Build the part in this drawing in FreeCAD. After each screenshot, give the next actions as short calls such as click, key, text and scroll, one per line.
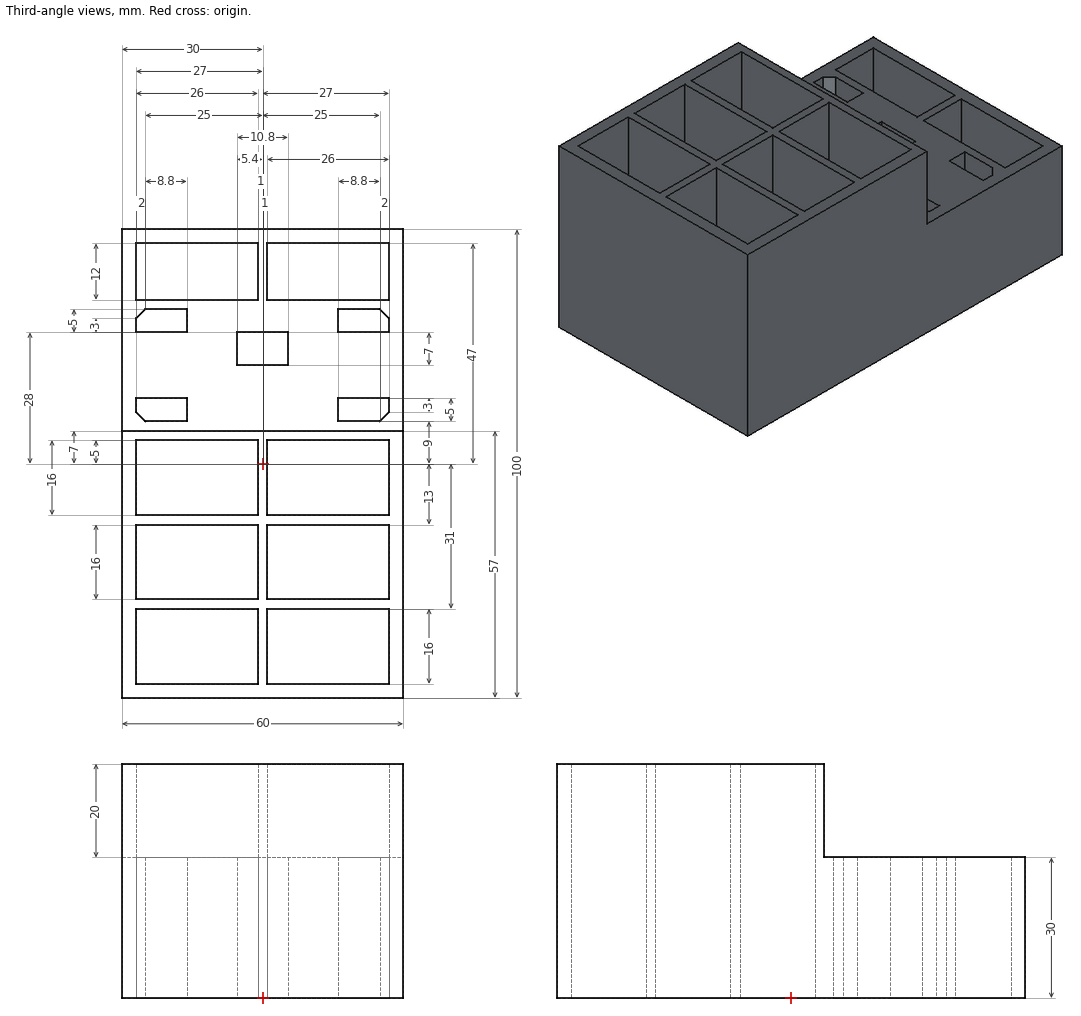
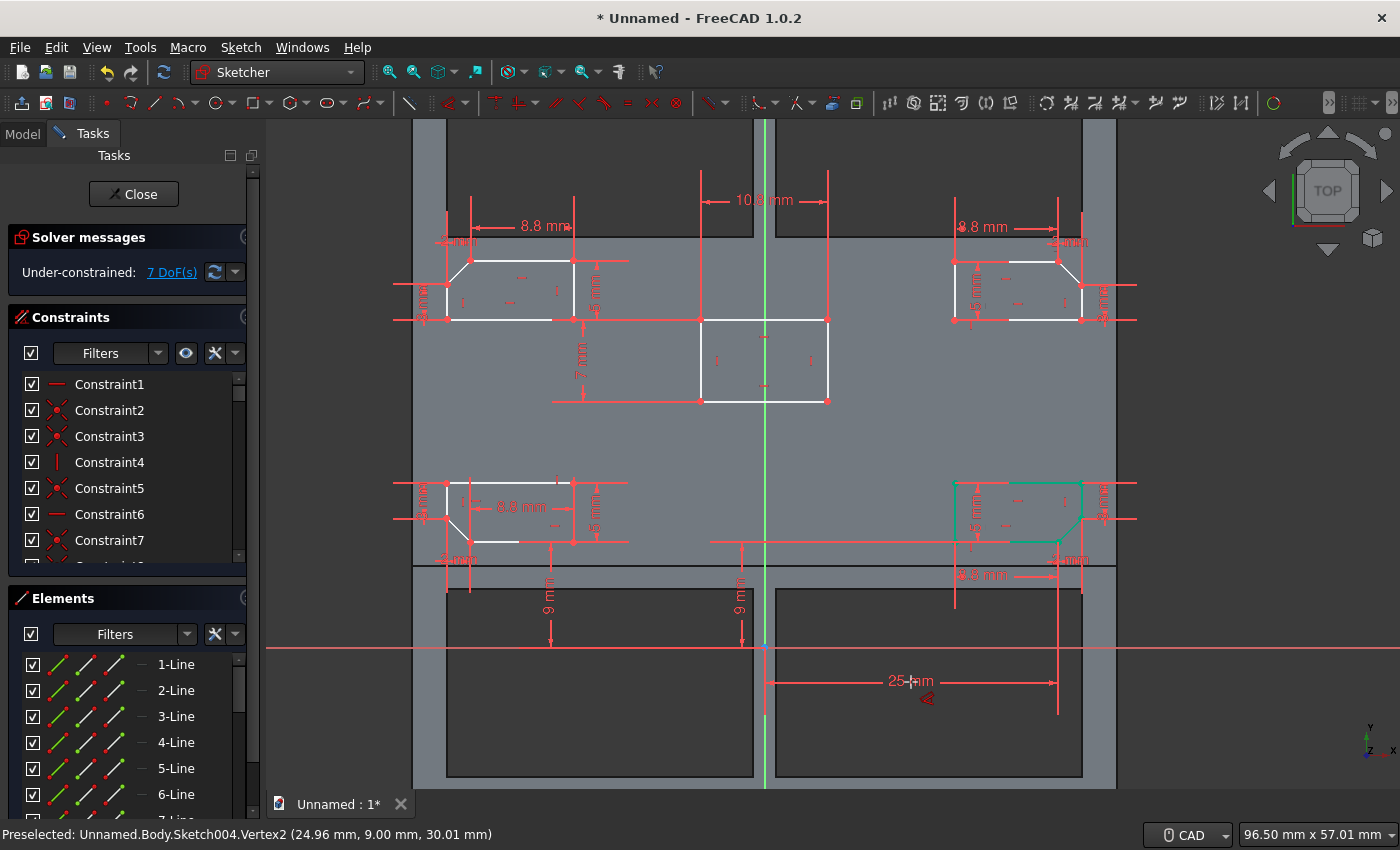
click(701, 320)
click(667, 484)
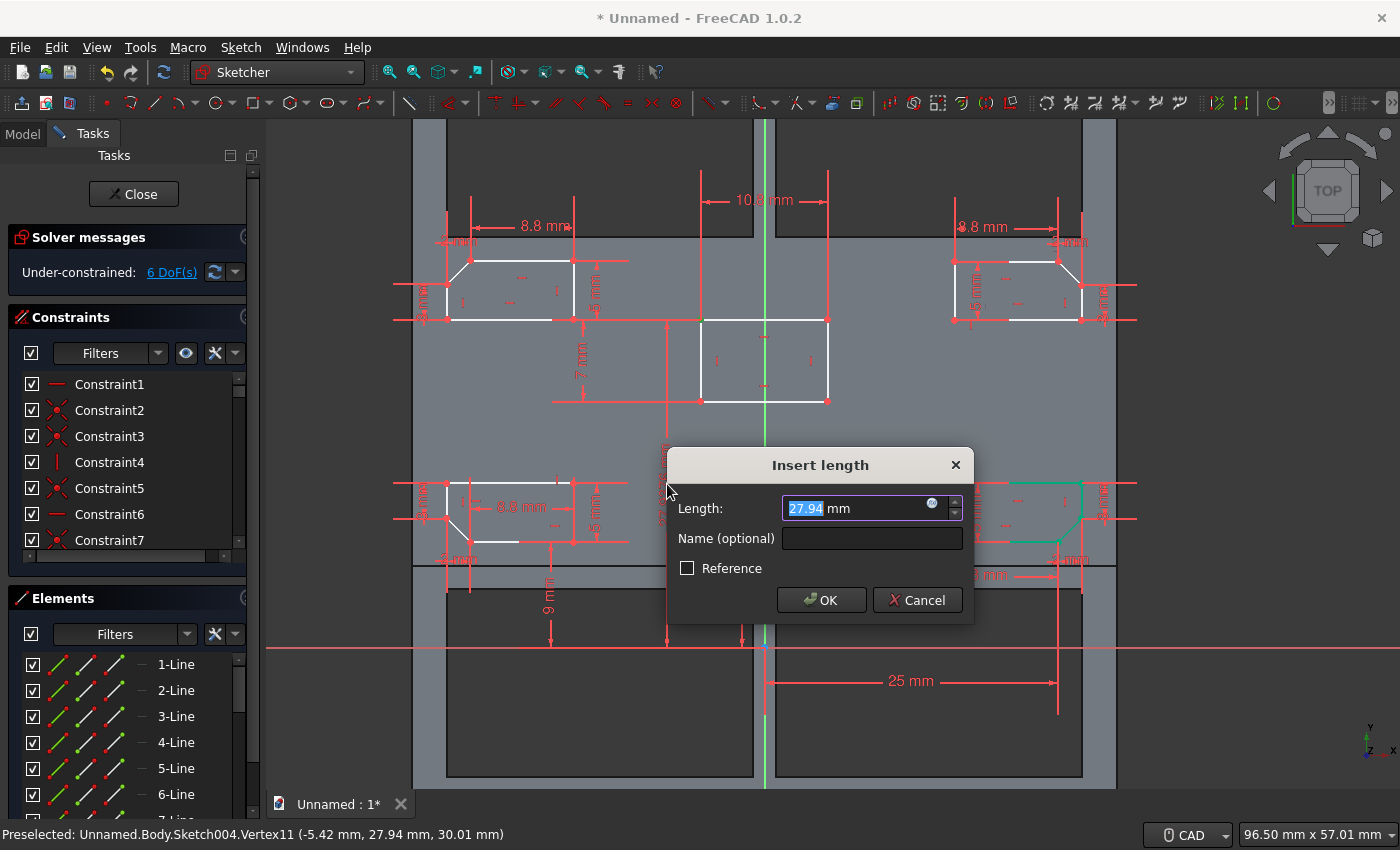
text(28)
key(Return)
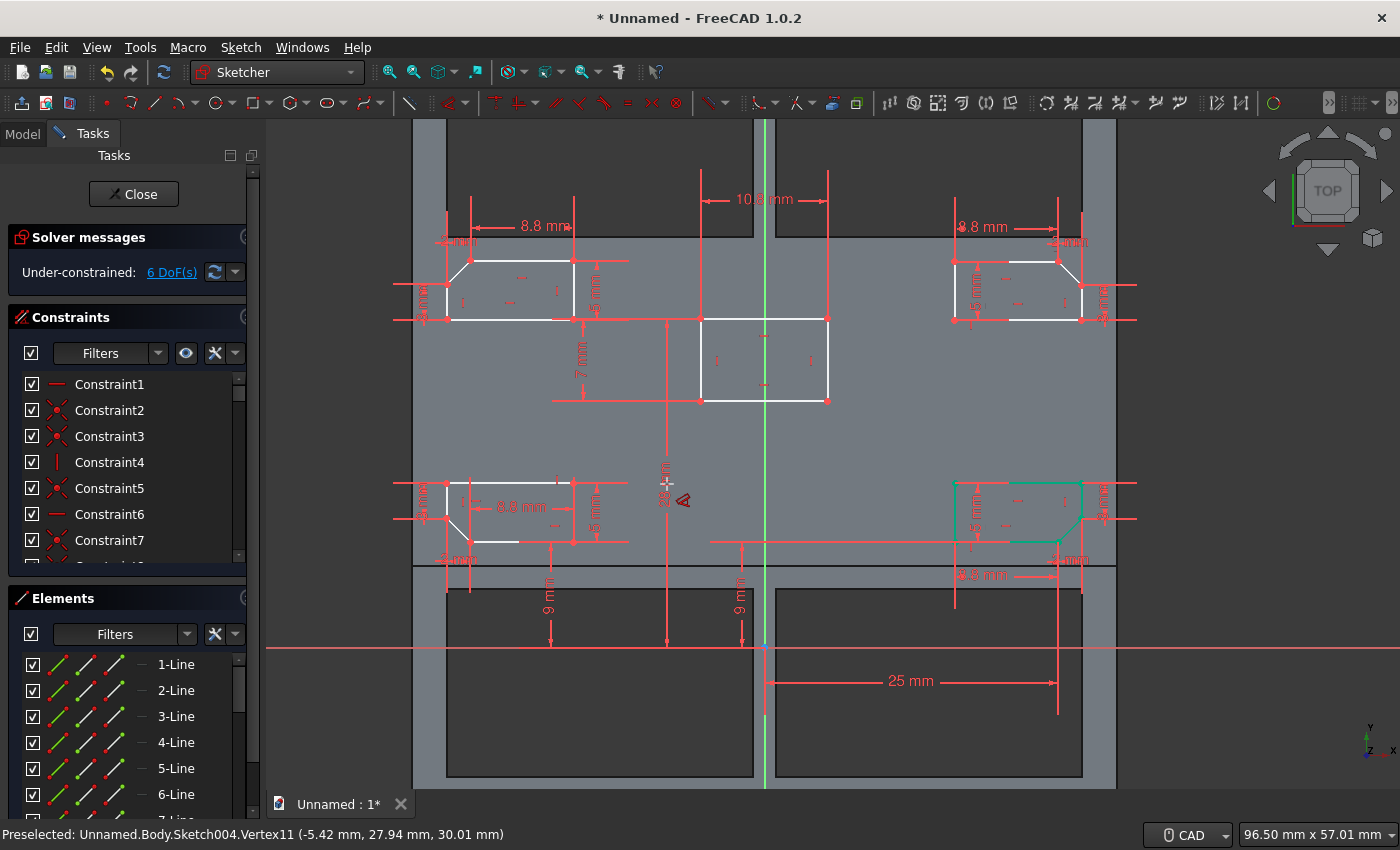
click(574, 320)
click(540, 408)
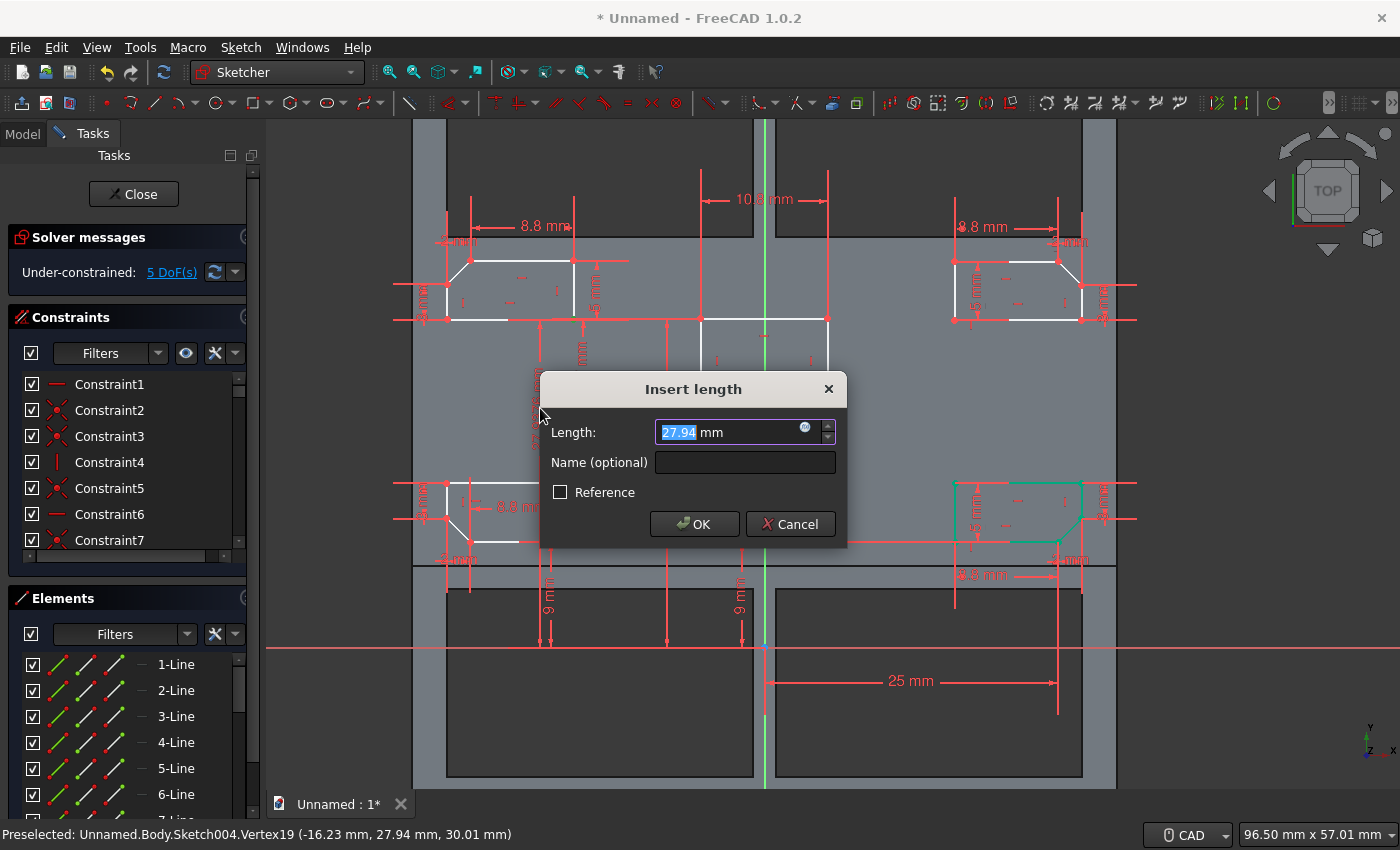
text(28)
key(Return)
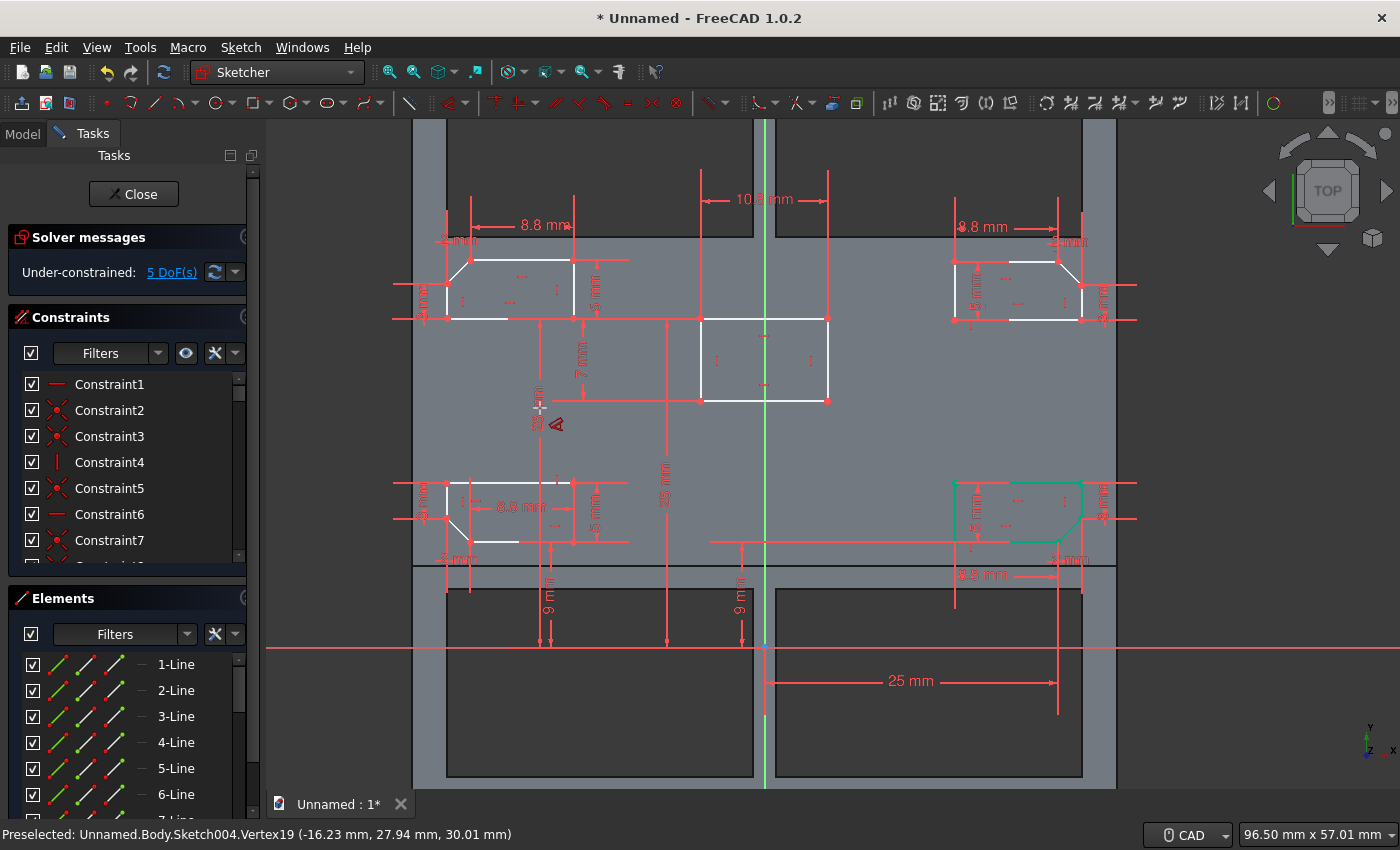
click(471, 260)
click(618, 682)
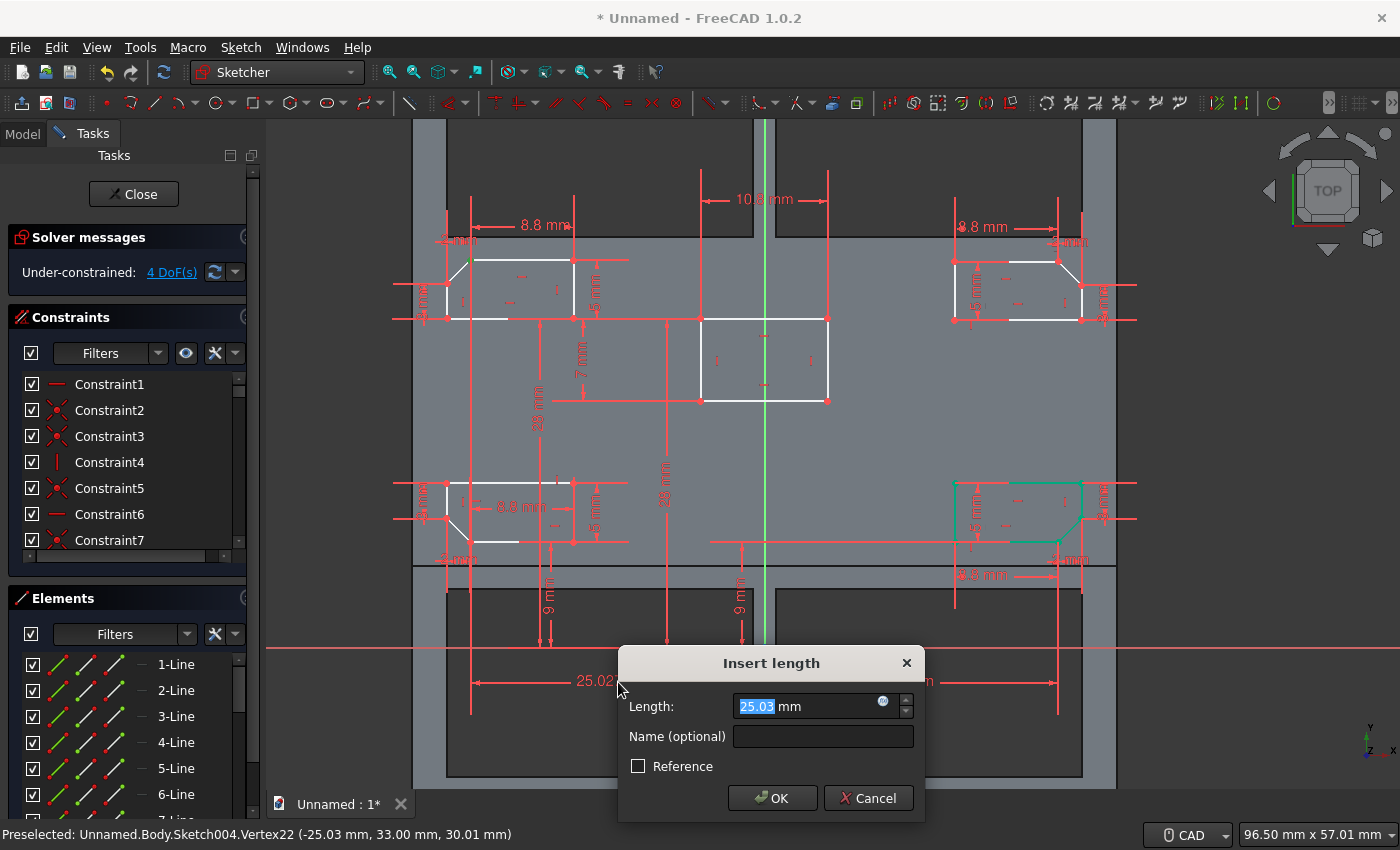
text(25)
key(Return)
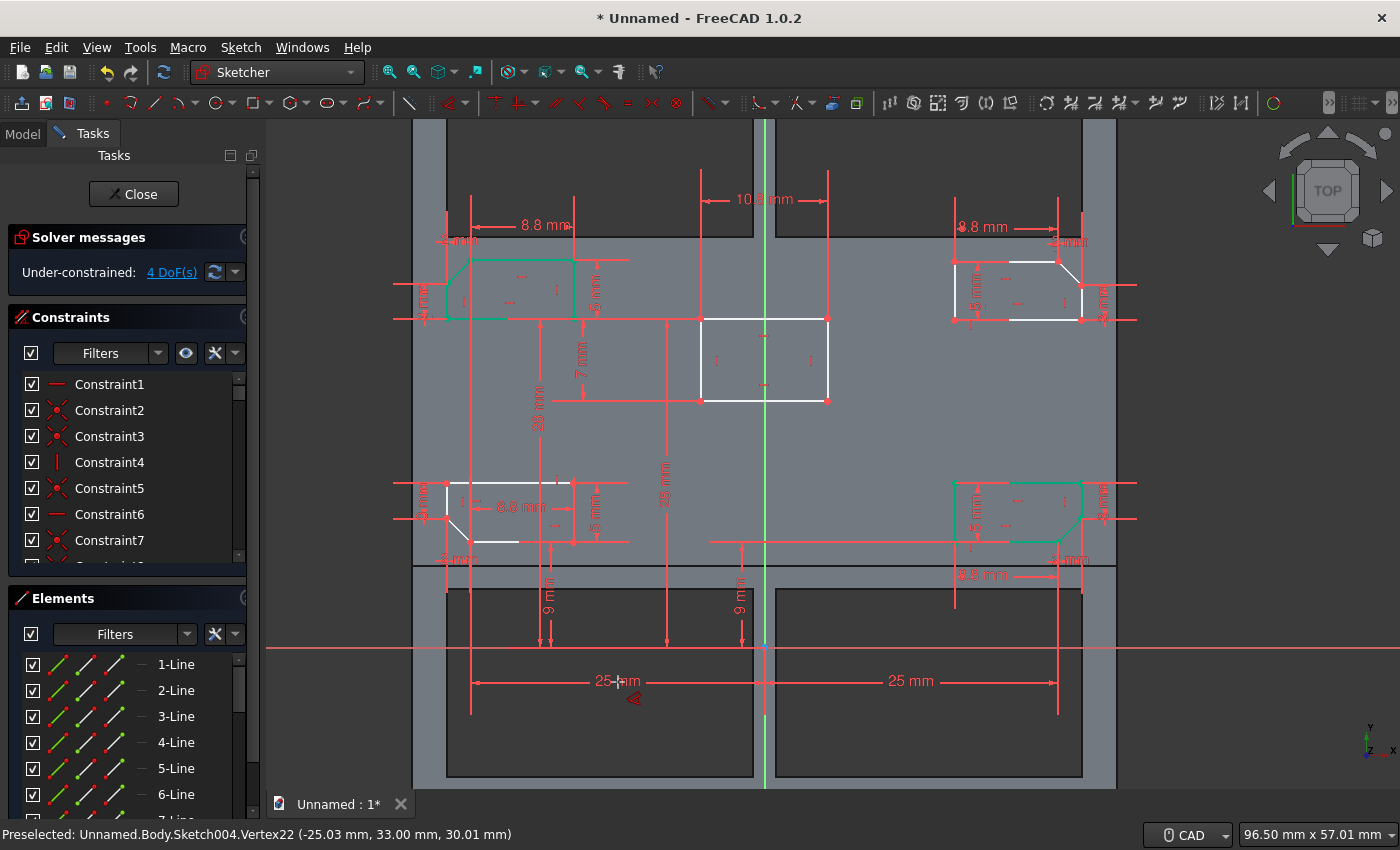
click(955, 320)
click(989, 409)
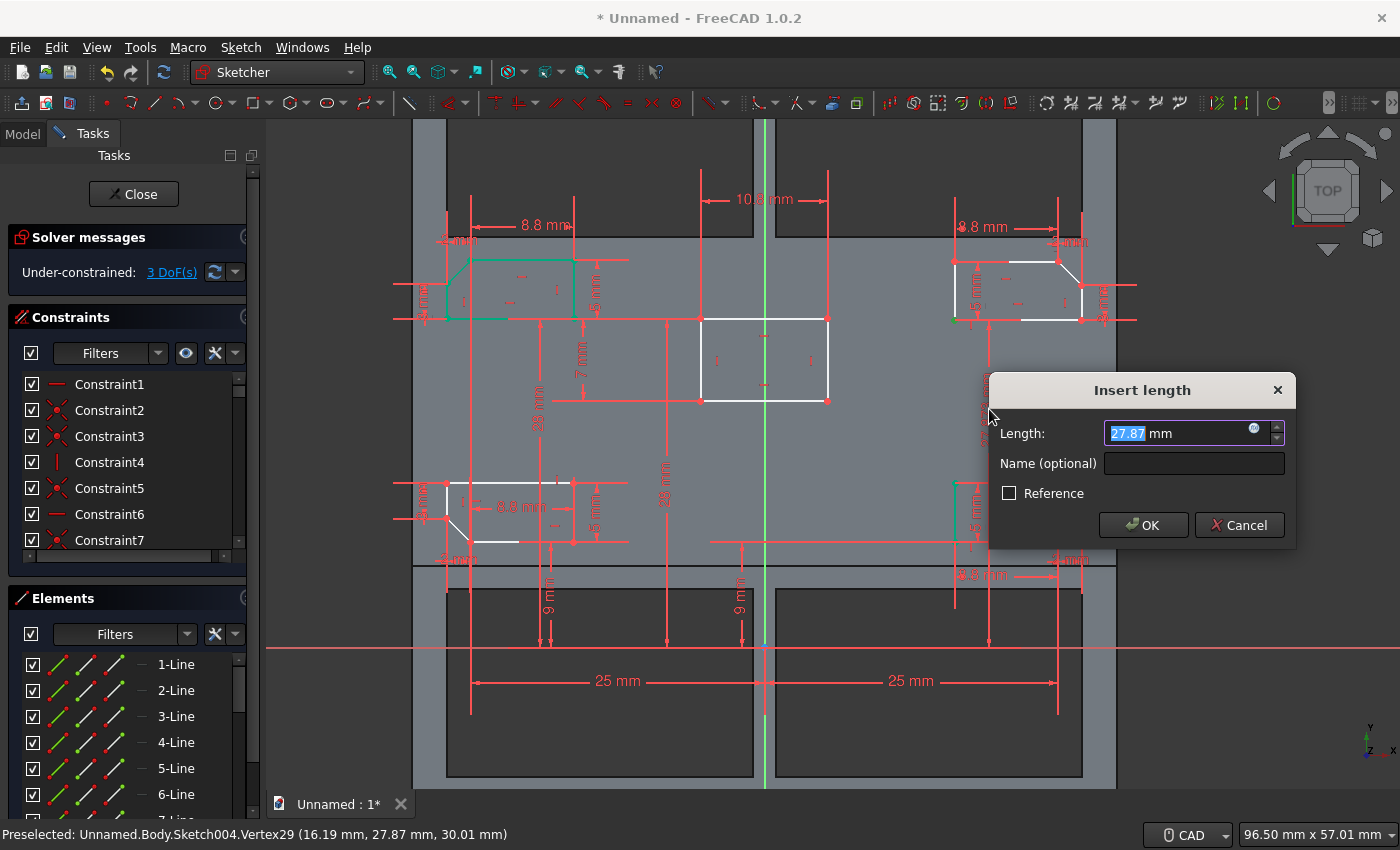
text(28)
key(Return)